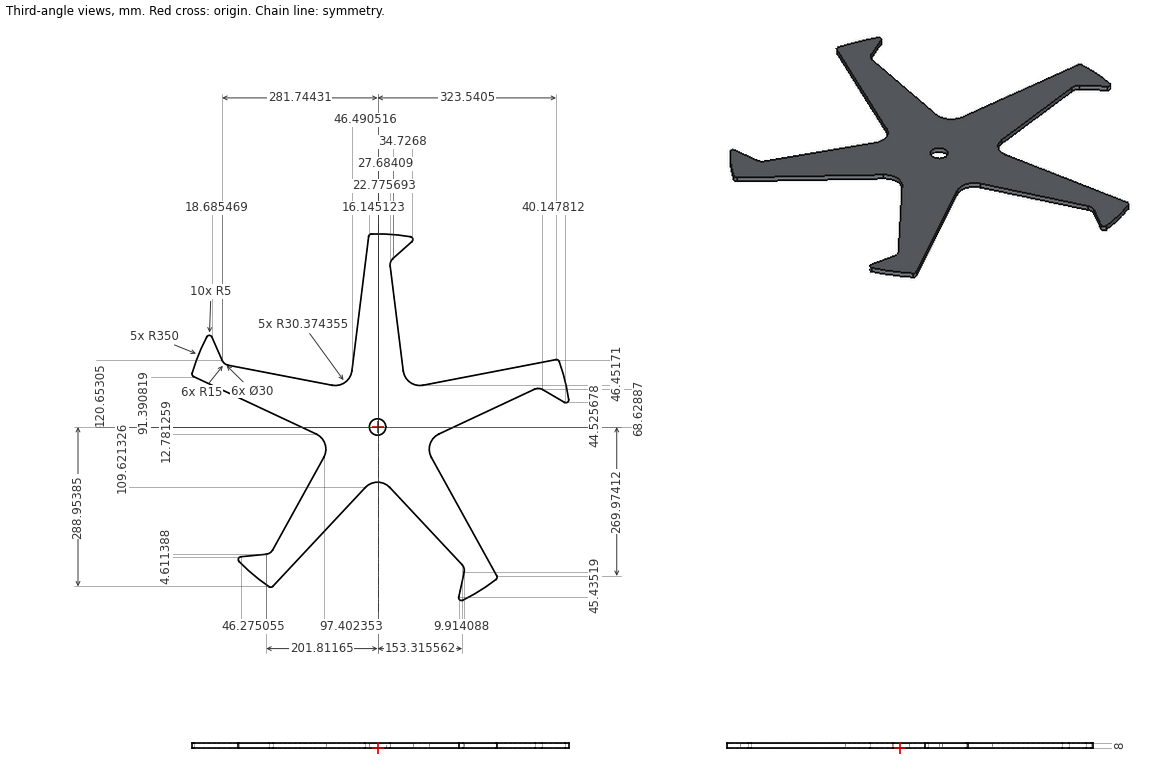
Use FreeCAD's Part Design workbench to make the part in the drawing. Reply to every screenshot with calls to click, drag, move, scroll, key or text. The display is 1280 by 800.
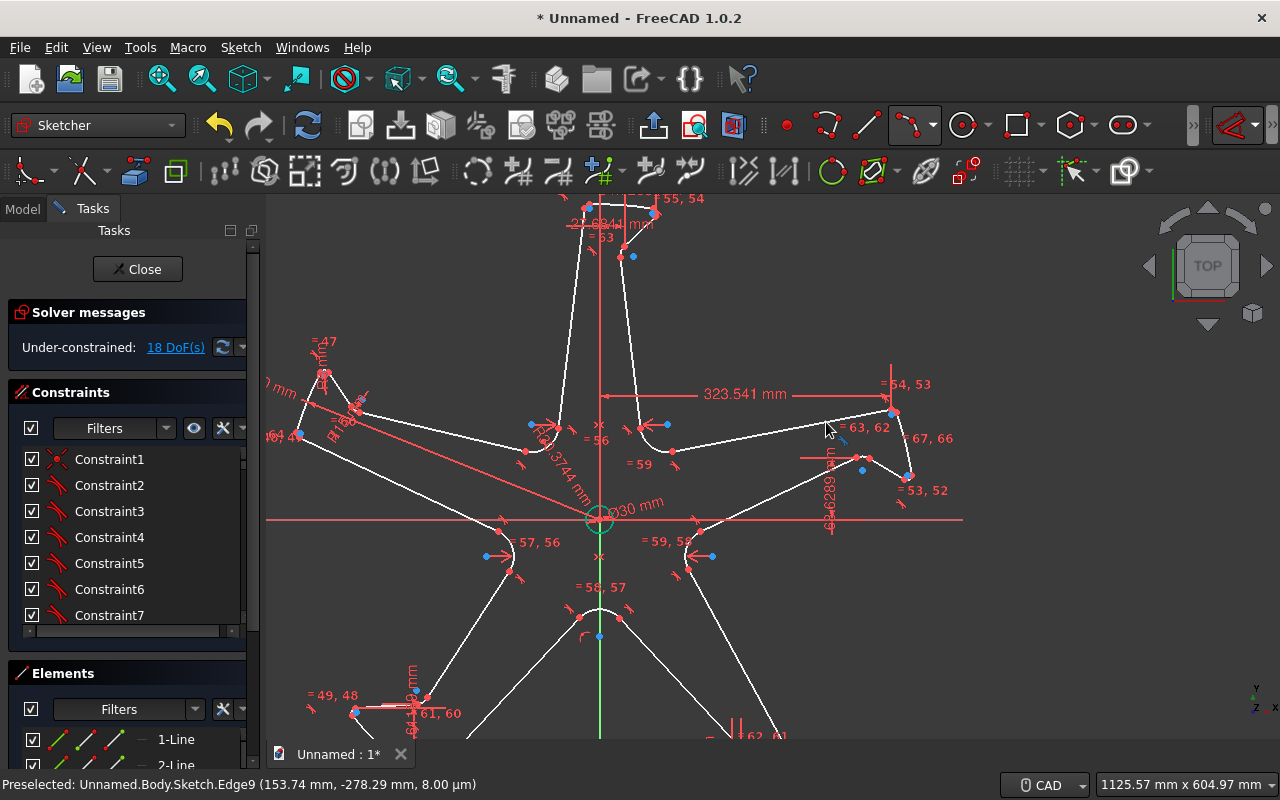
click(826, 422)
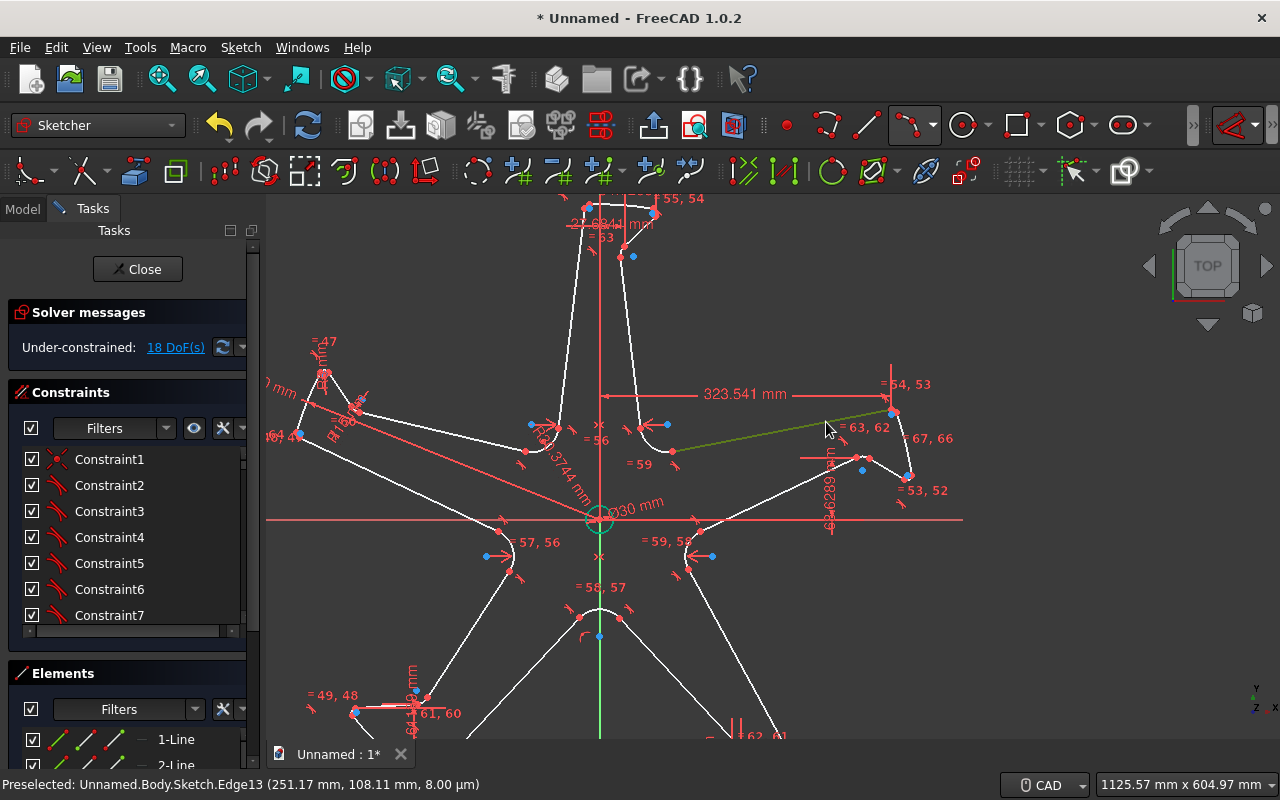
key(i)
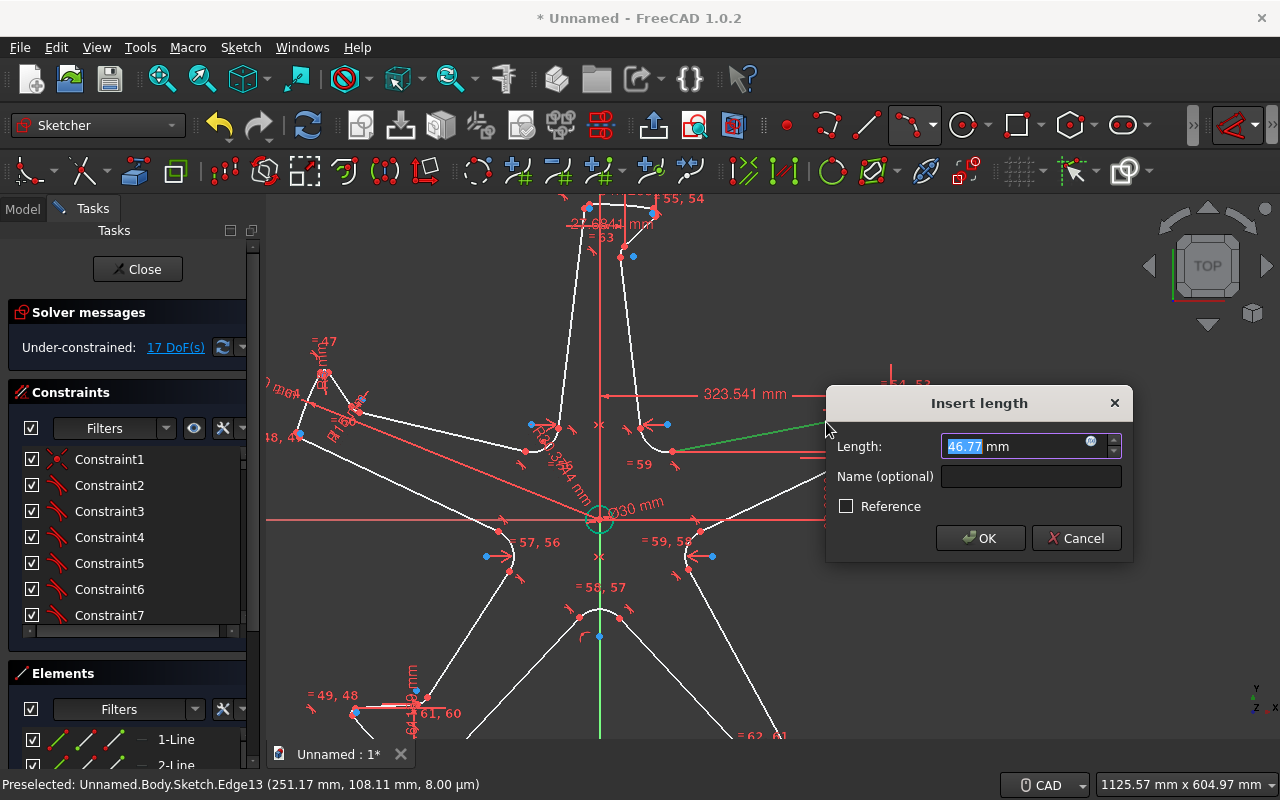
text(46.45171)
key(Return)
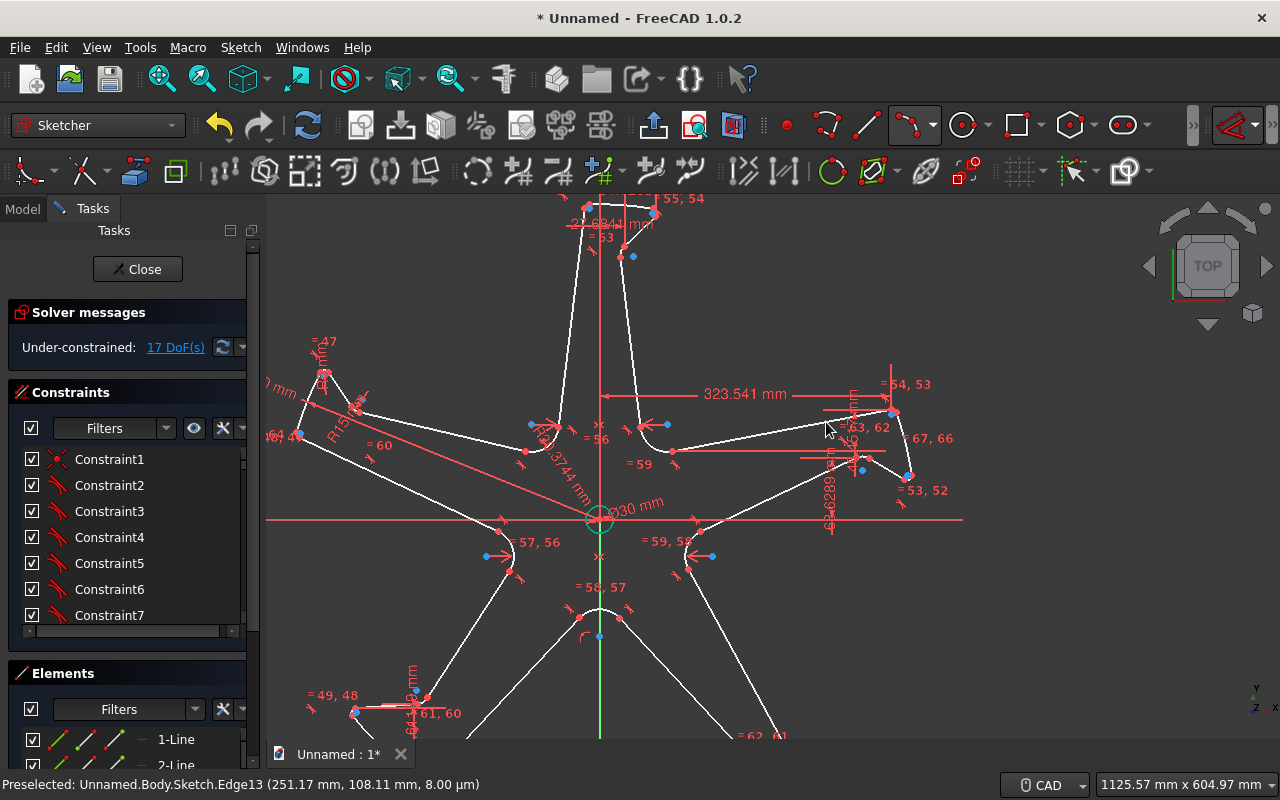
scroll(826, 421, down, 3)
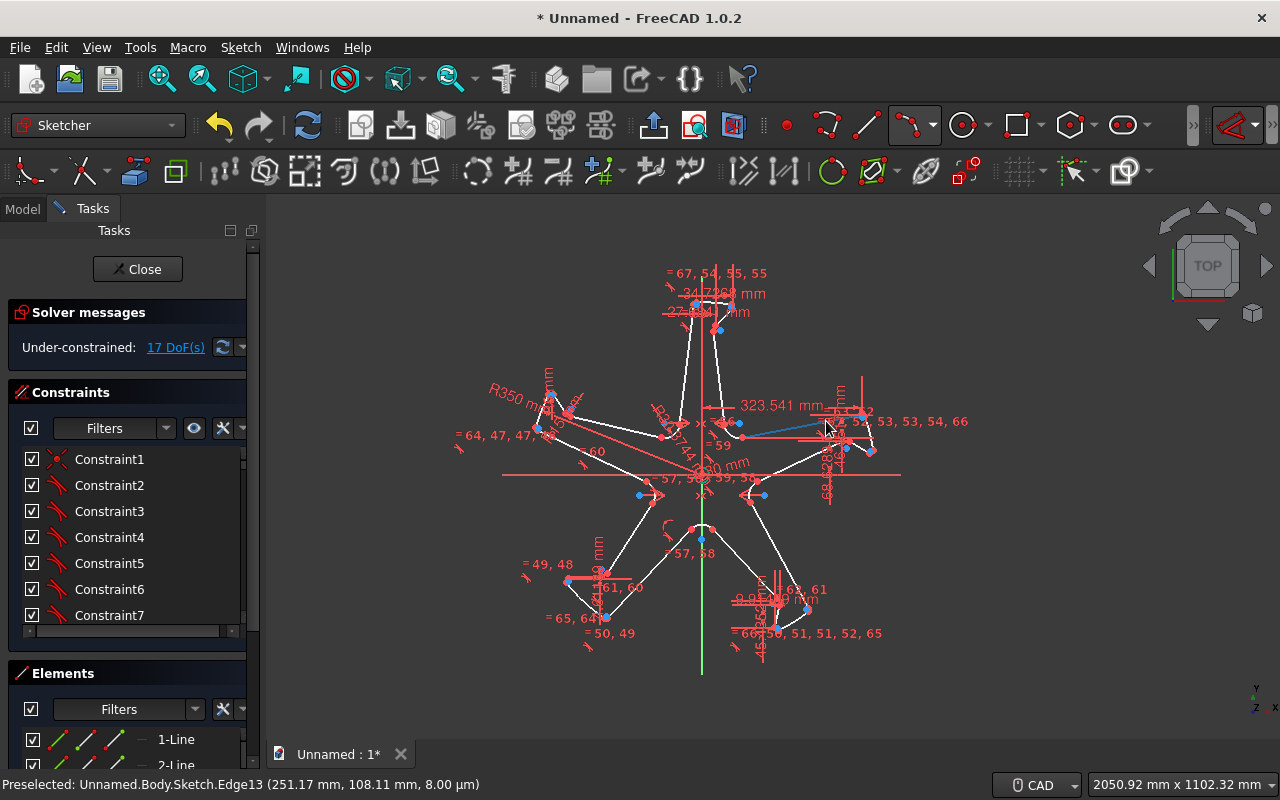
scroll(694, 305, up, 9)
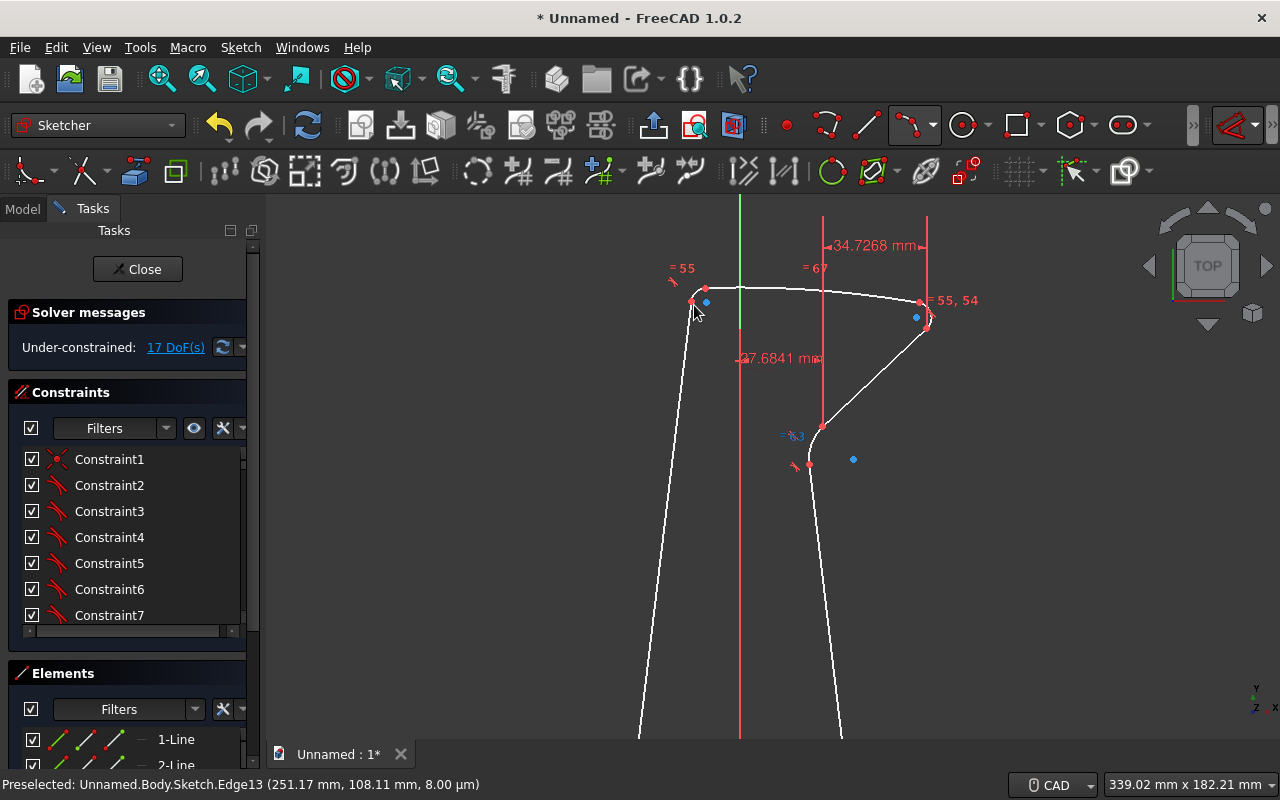
click(692, 301)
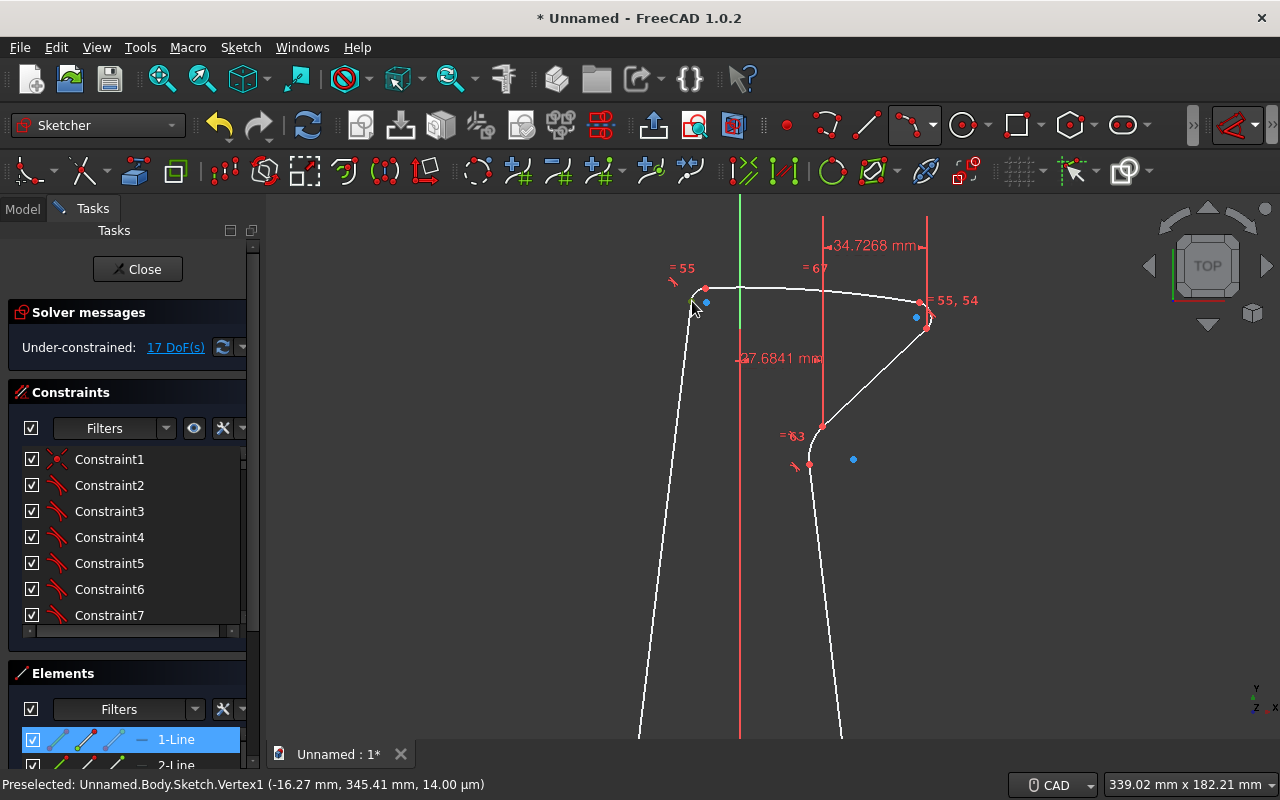
key(l)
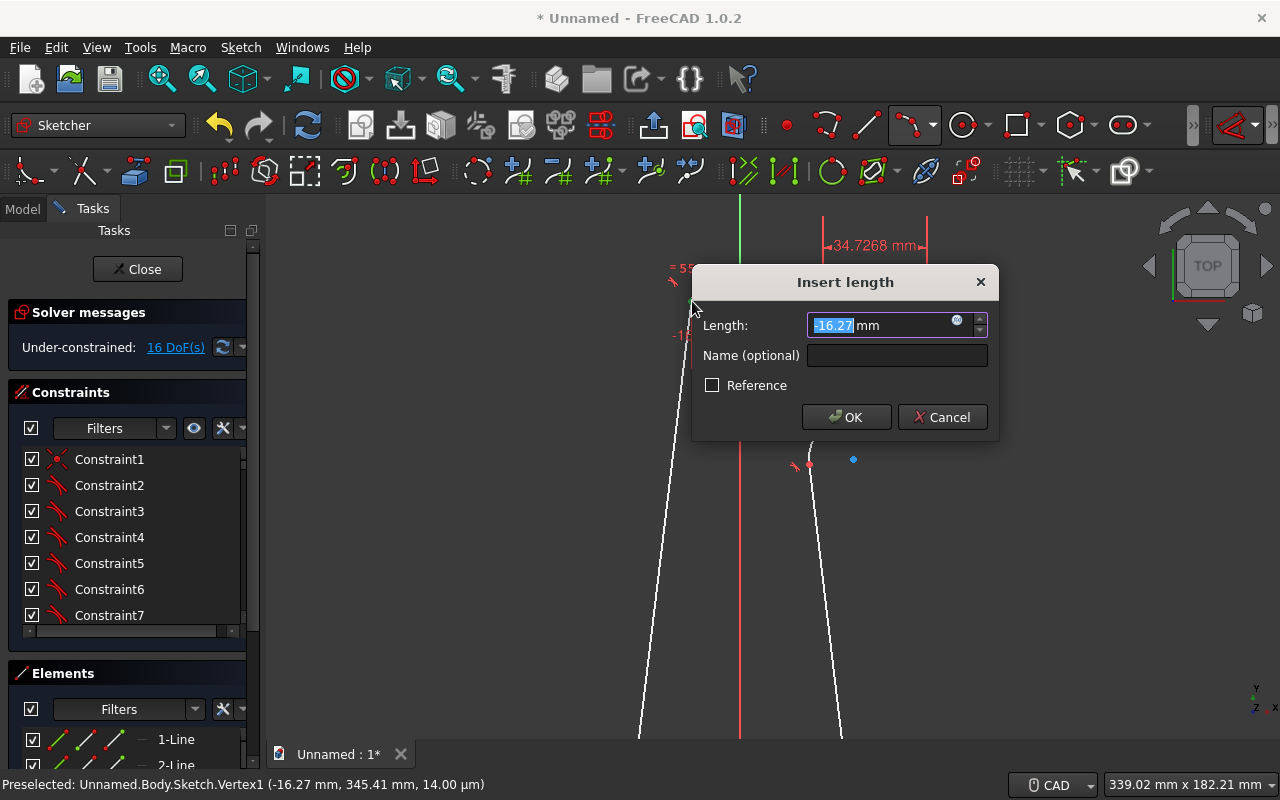
text(-16.145123)
key(Return)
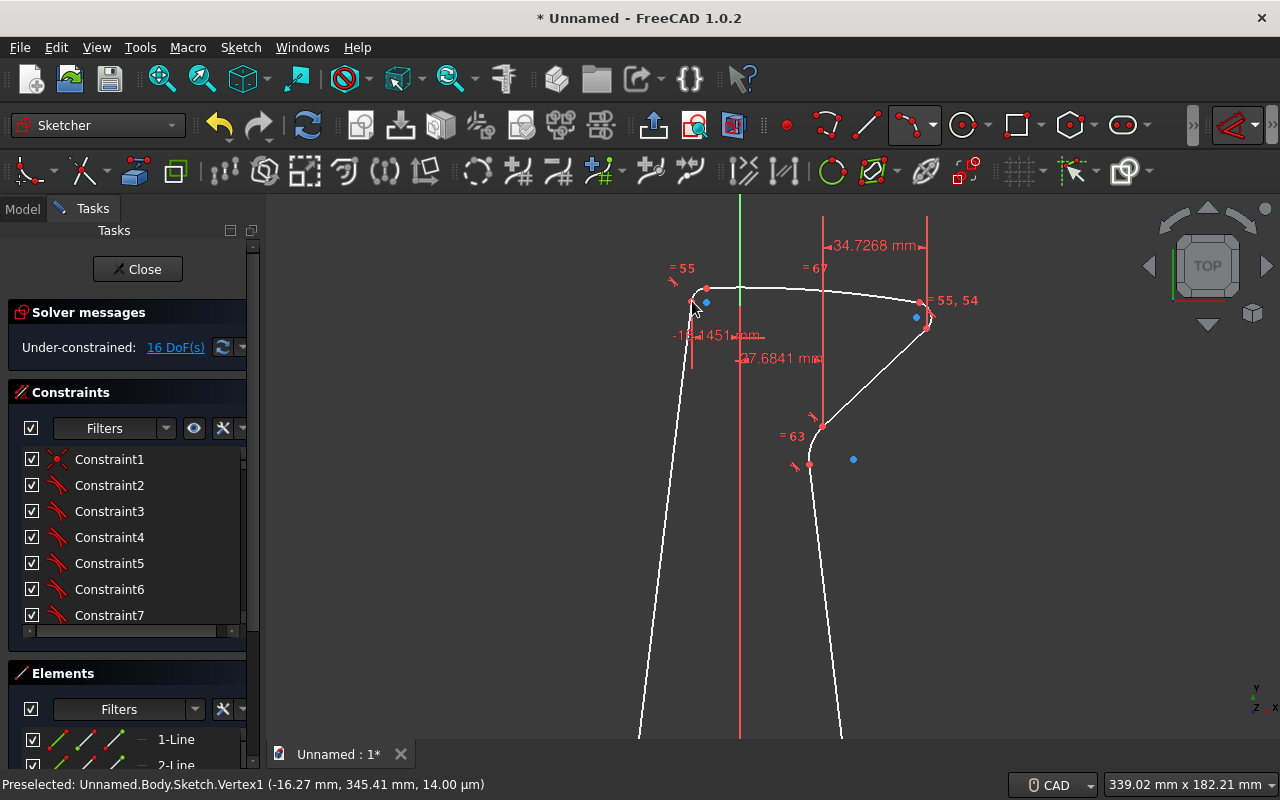
scroll(694, 305, down, 9)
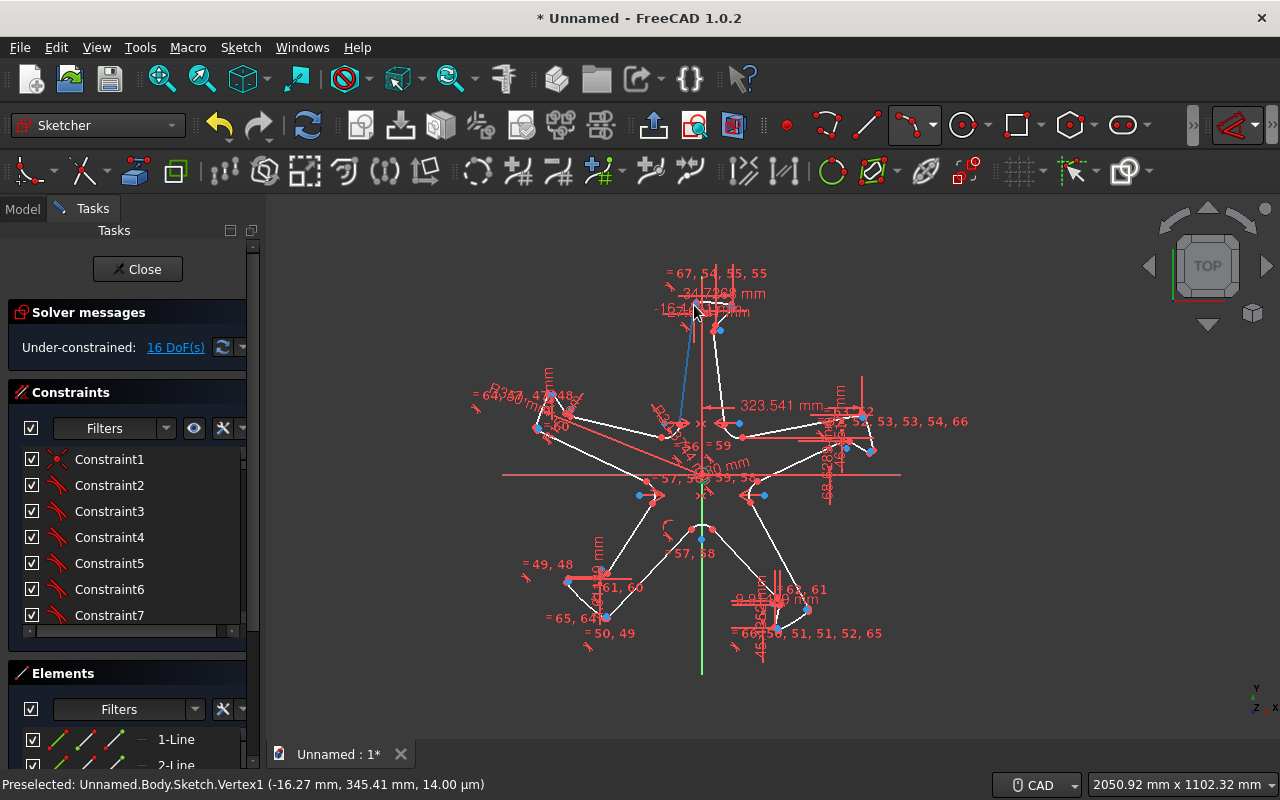
scroll(679, 425, up, 3)